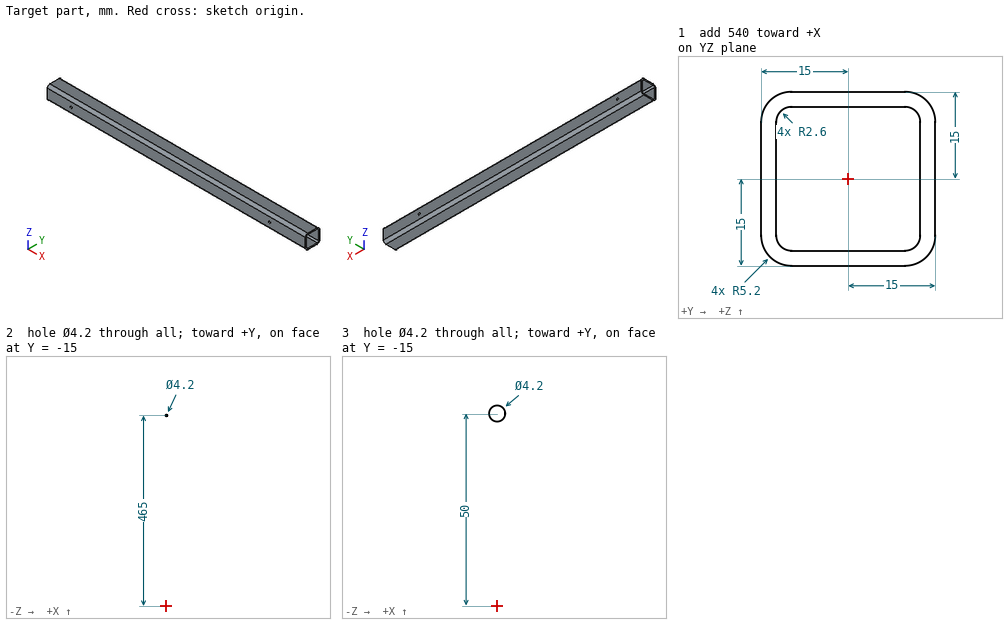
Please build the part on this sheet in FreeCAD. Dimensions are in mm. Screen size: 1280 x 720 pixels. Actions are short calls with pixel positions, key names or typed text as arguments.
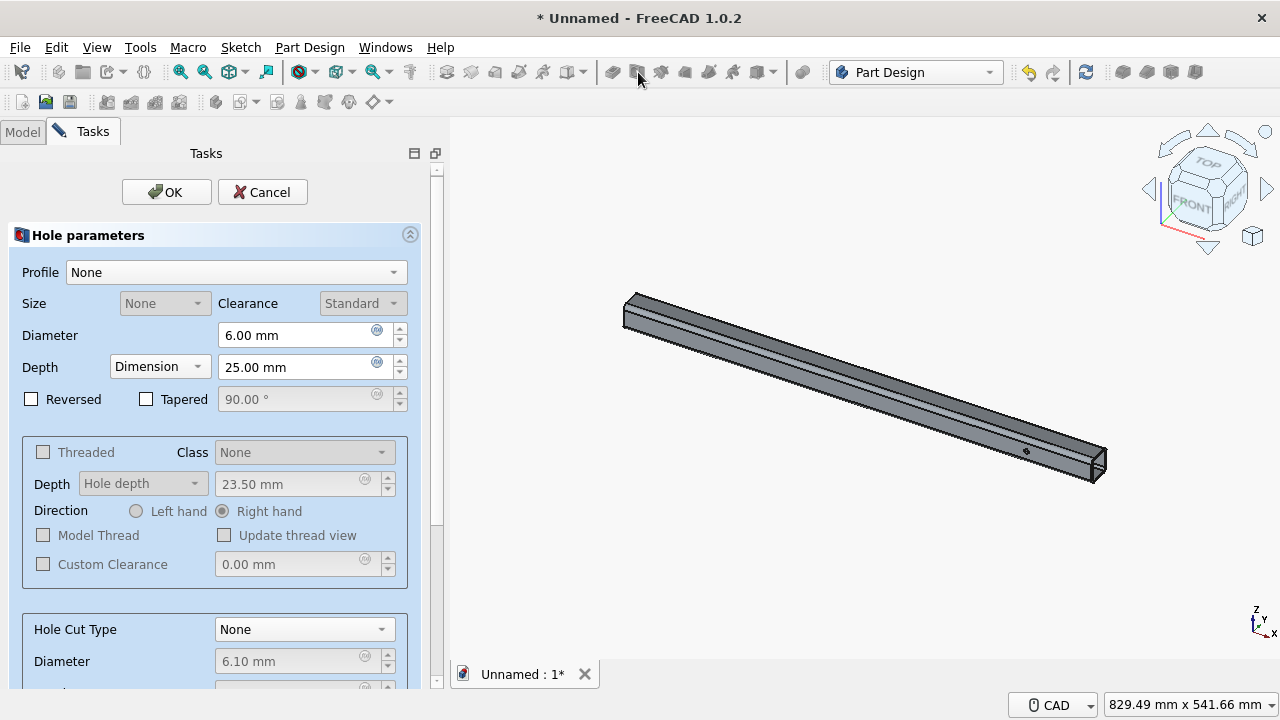
triple_click(305, 335)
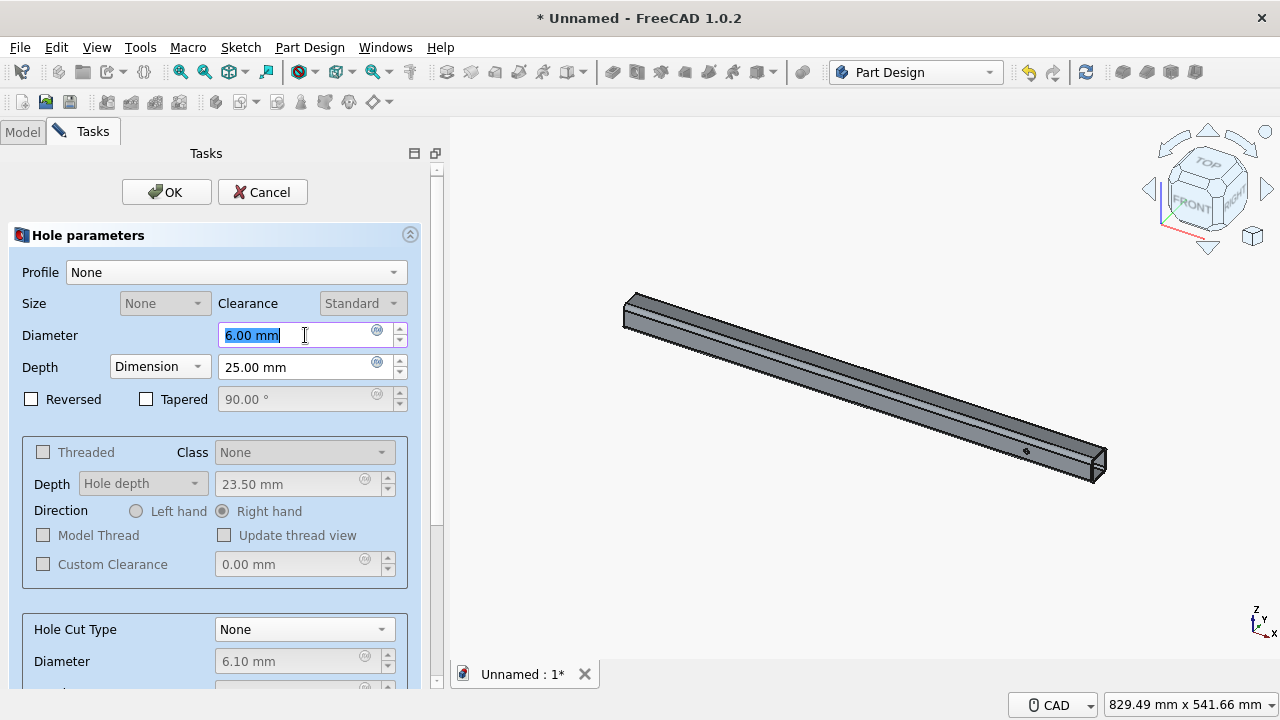
text(4.2)
key(Tab)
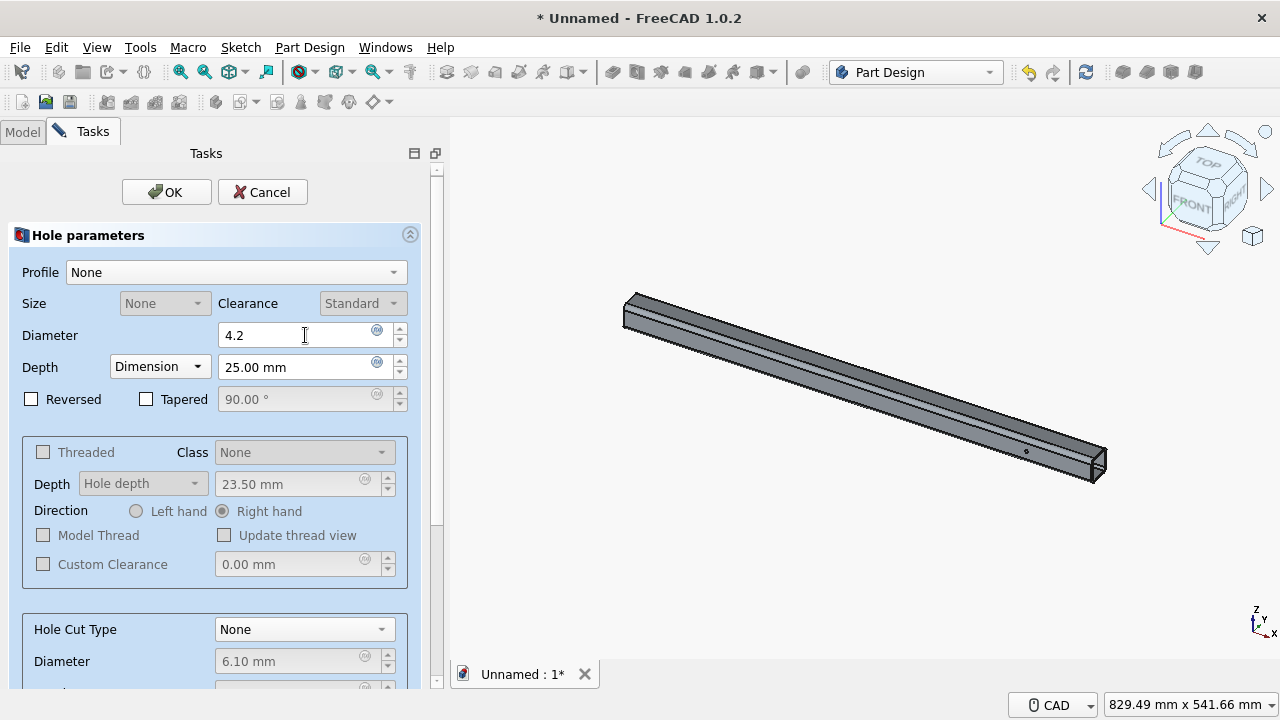
click(161, 366)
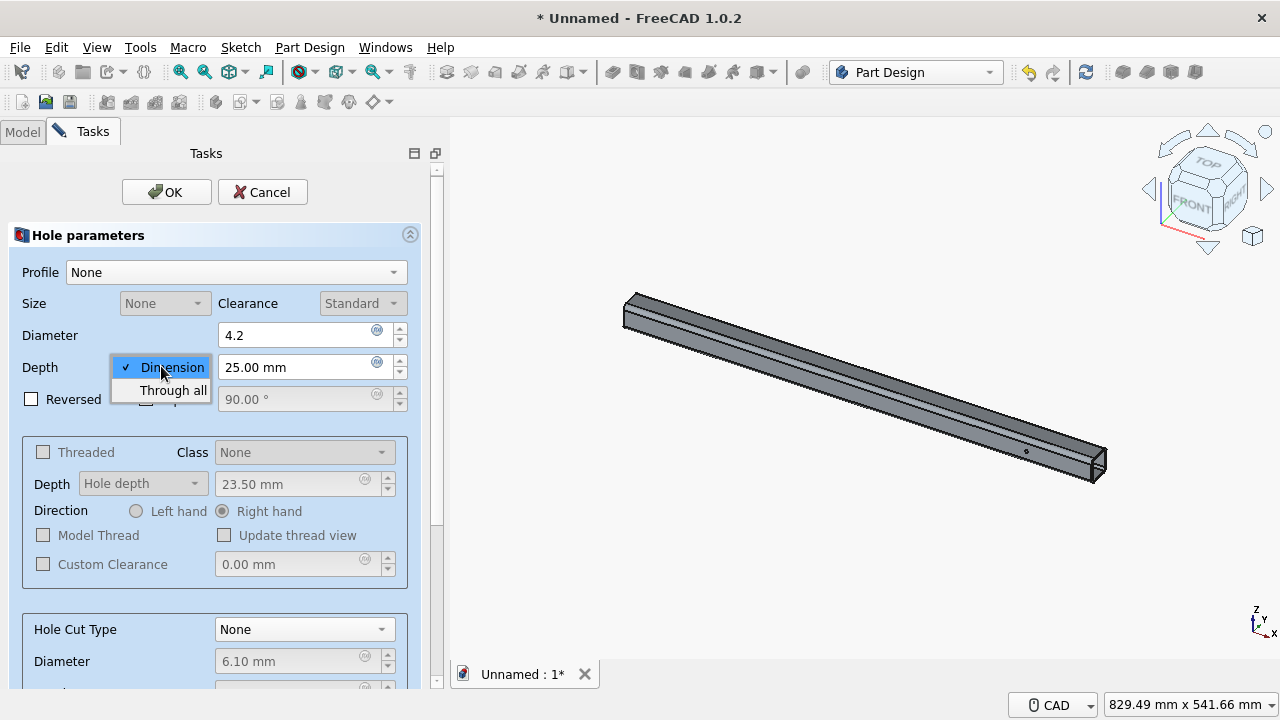
click(160, 390)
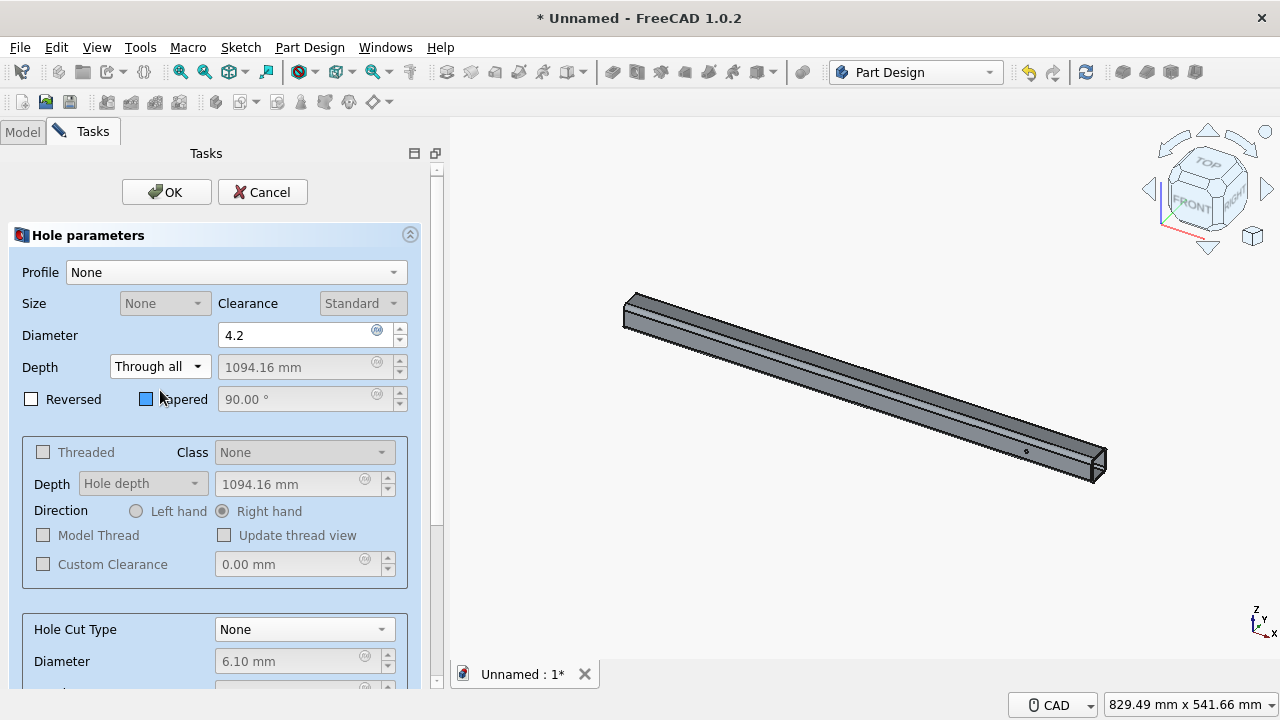
click(167, 192)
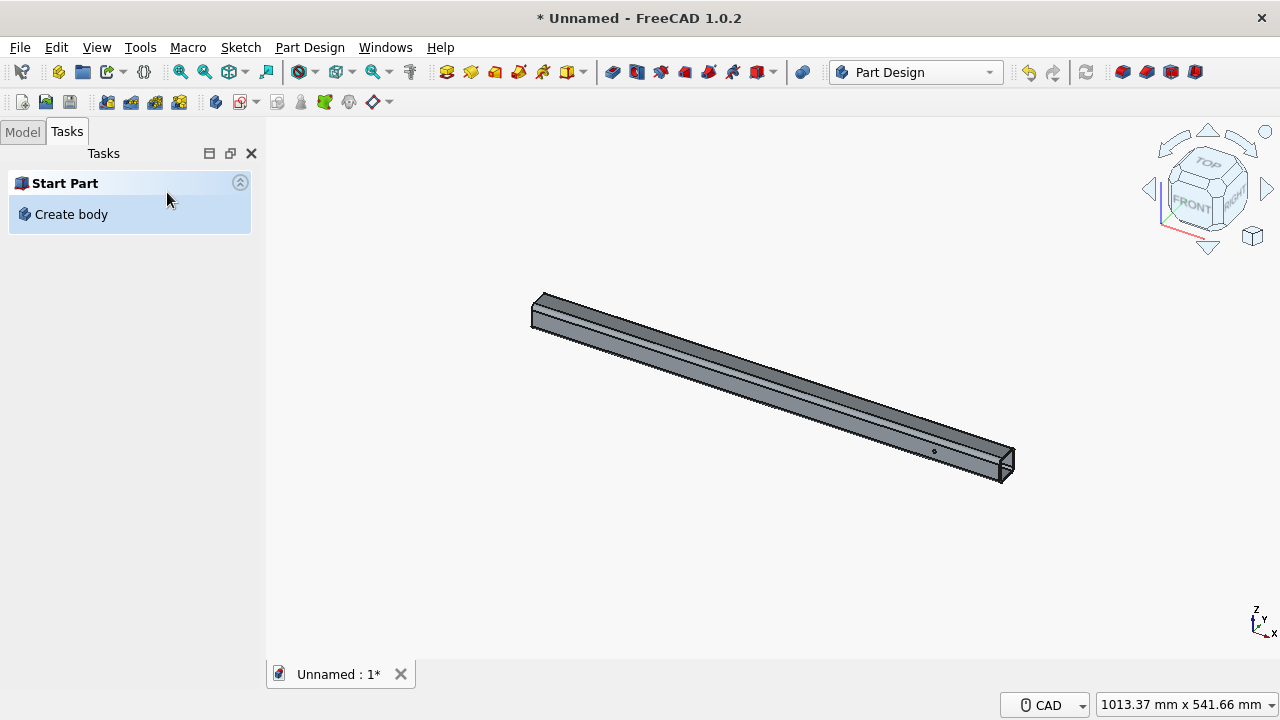
click(966, 463)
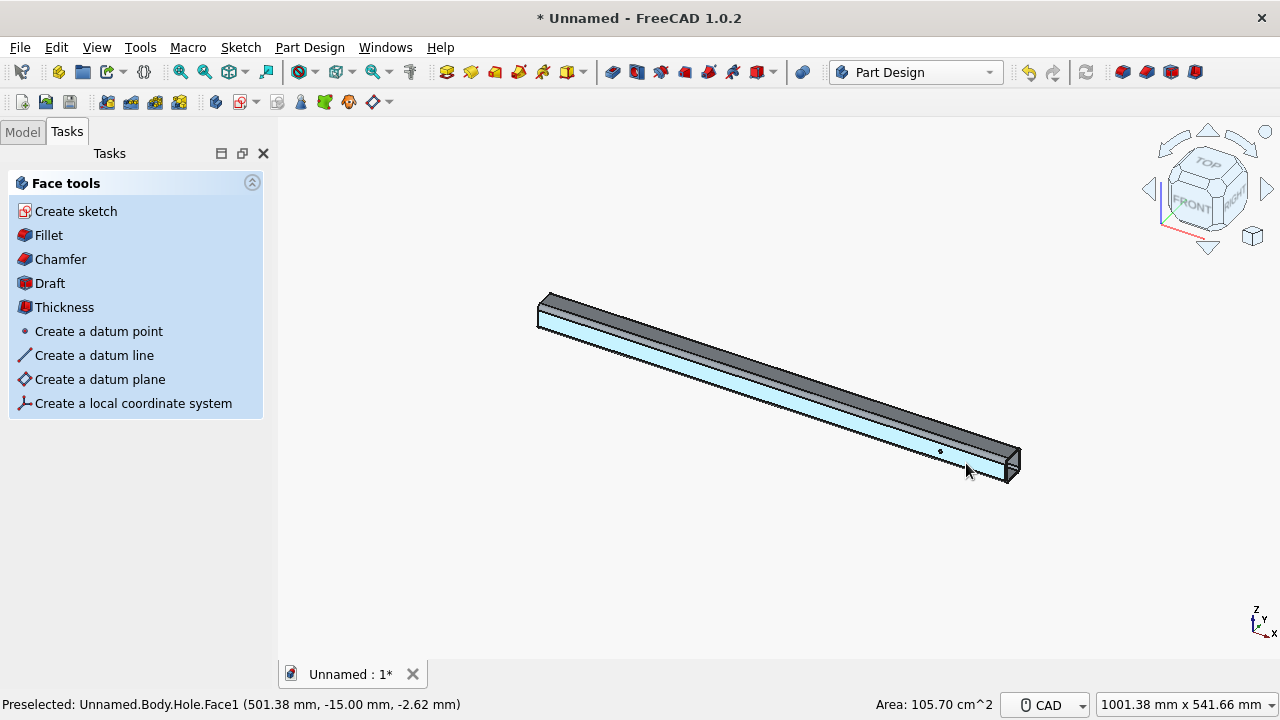
click(240, 102)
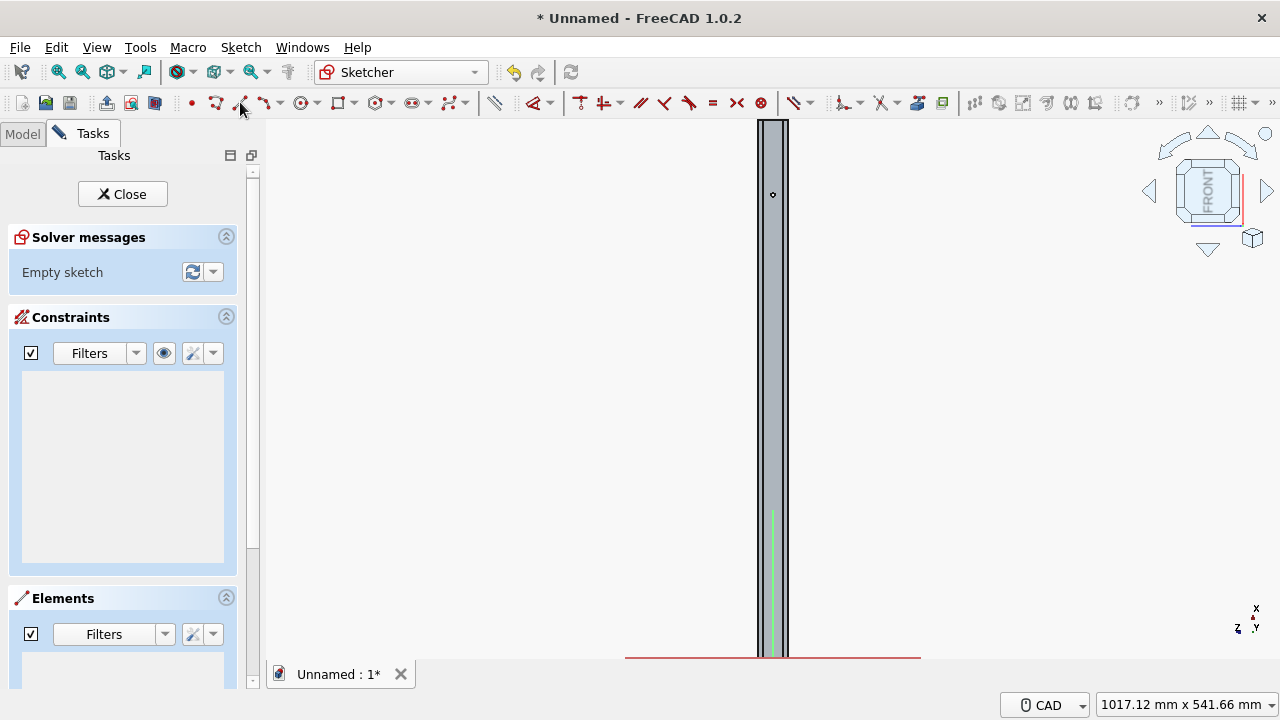
scroll(777, 620, up, 15)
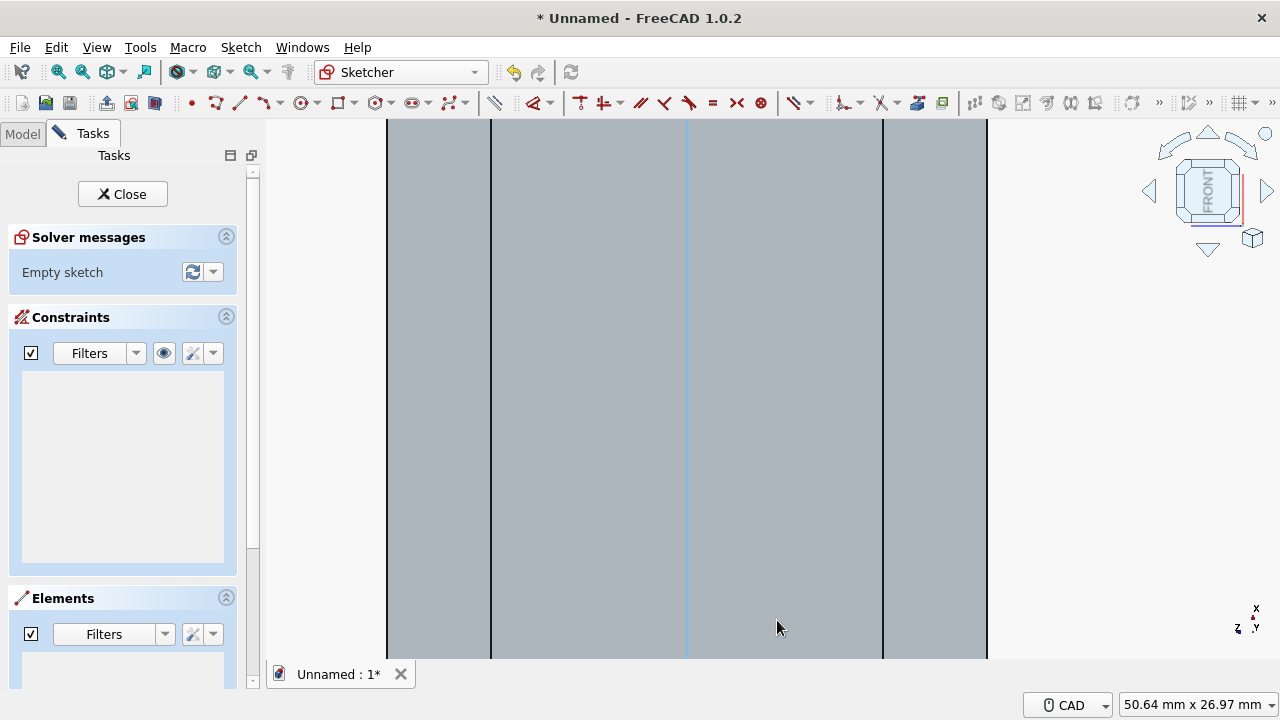
scroll(681, 361, up, 7)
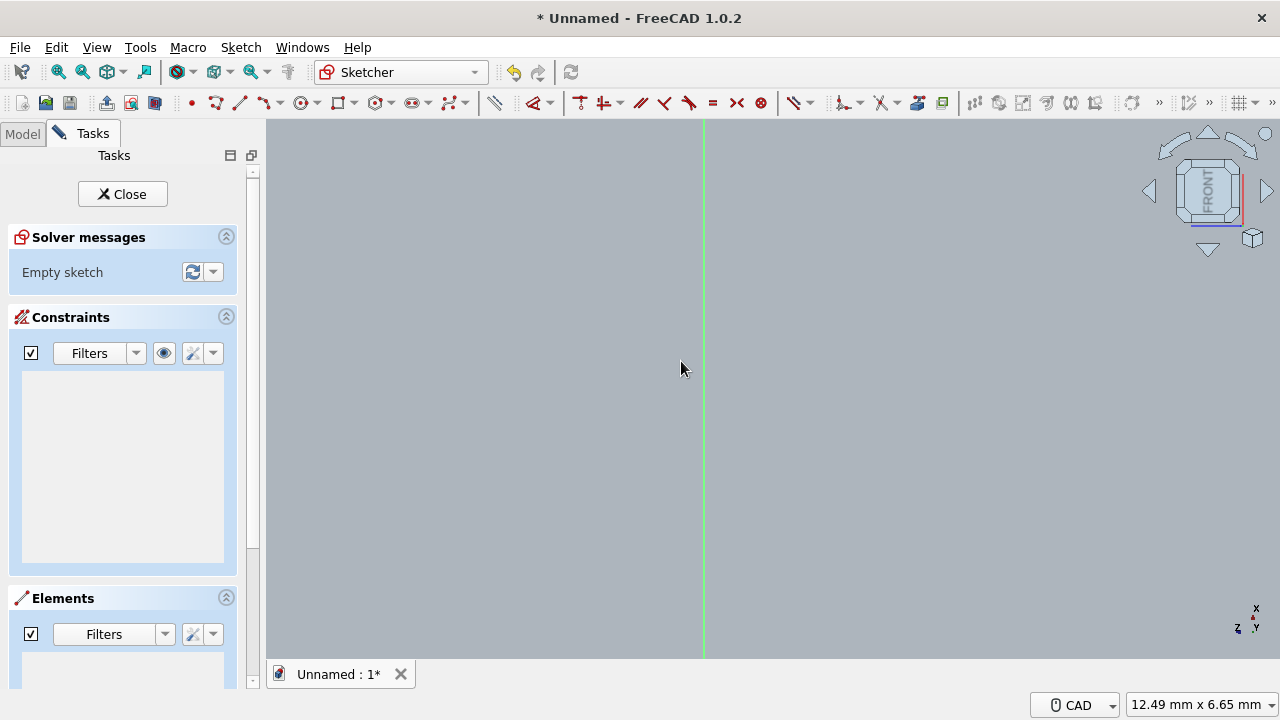
click(302, 104)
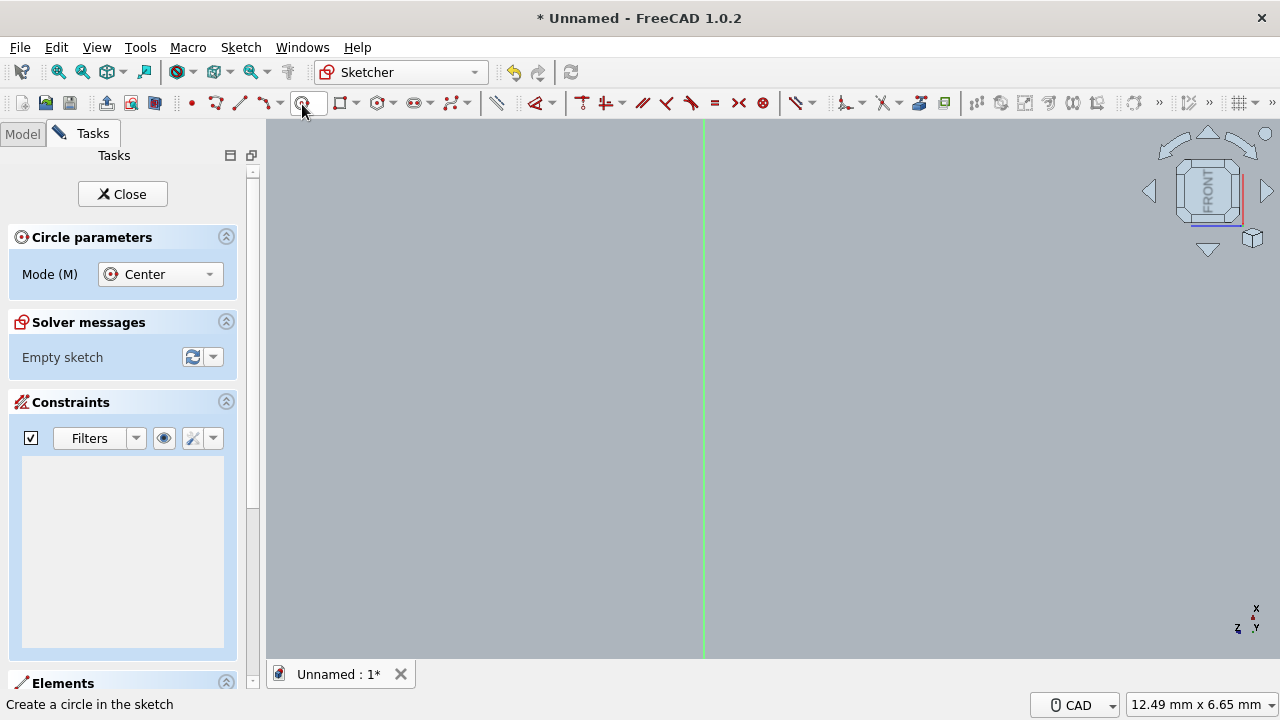
click(704, 387)
click(825, 266)
key(Escape)